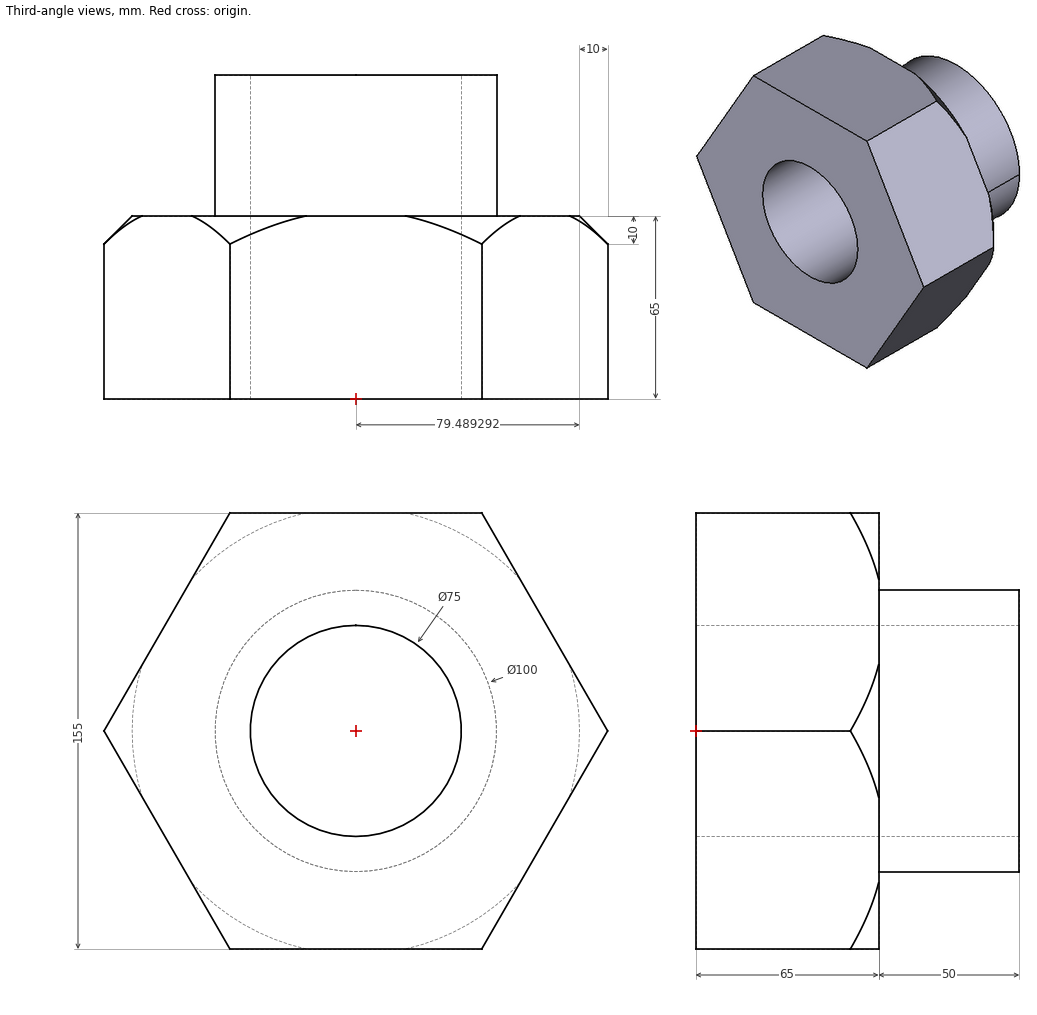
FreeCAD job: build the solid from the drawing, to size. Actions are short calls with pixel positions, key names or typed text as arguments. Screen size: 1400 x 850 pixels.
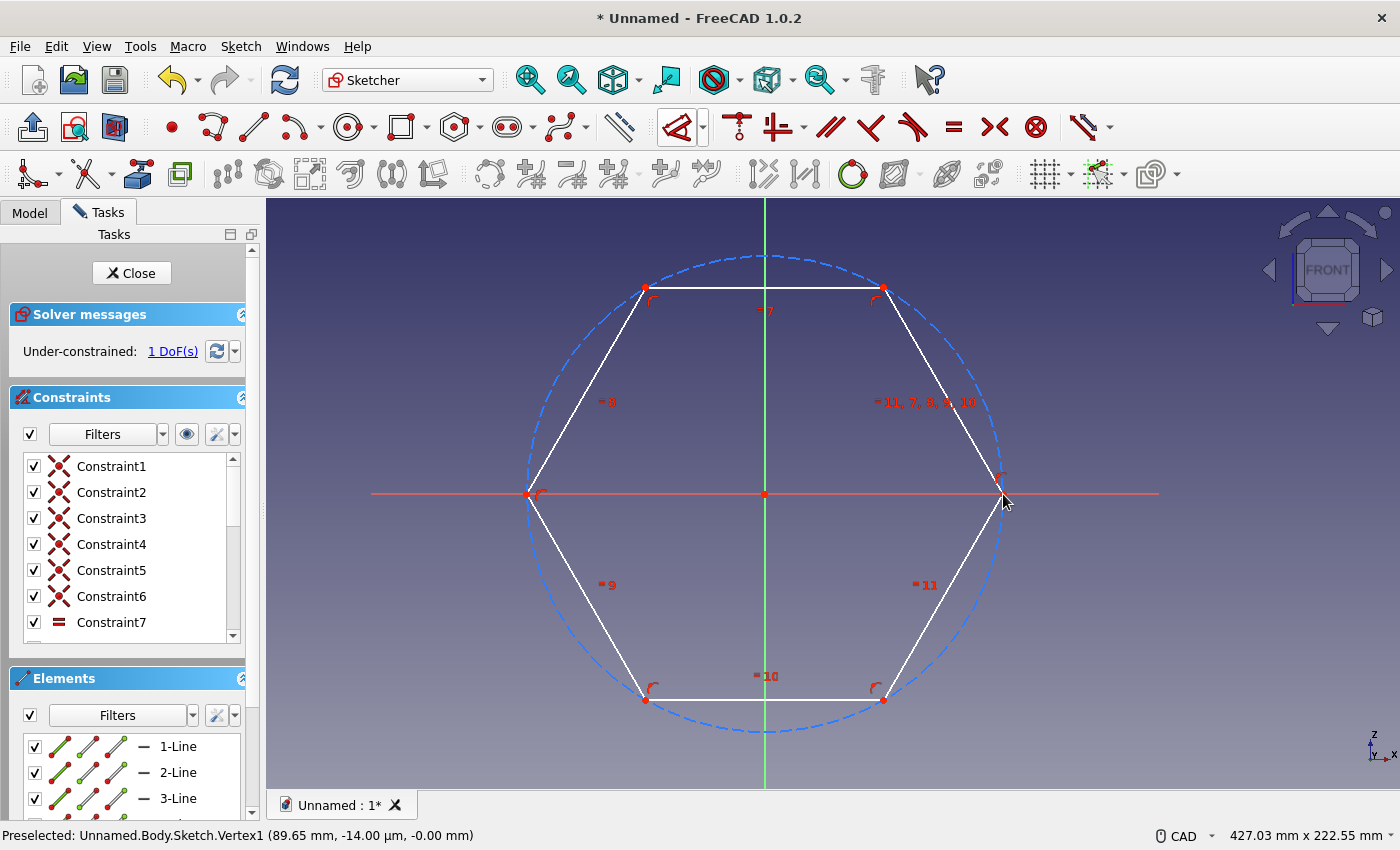
click(646, 700)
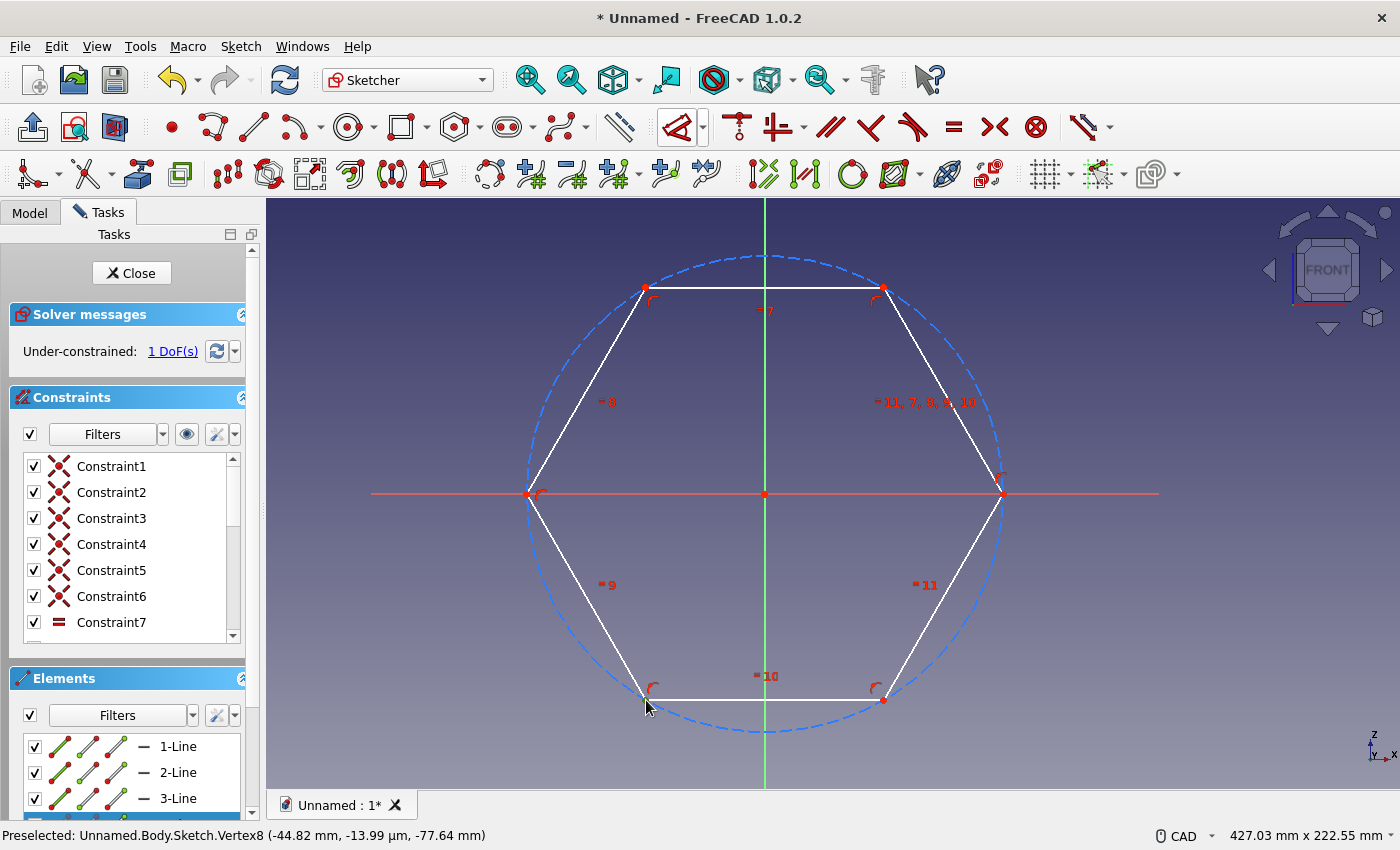
click(884, 288)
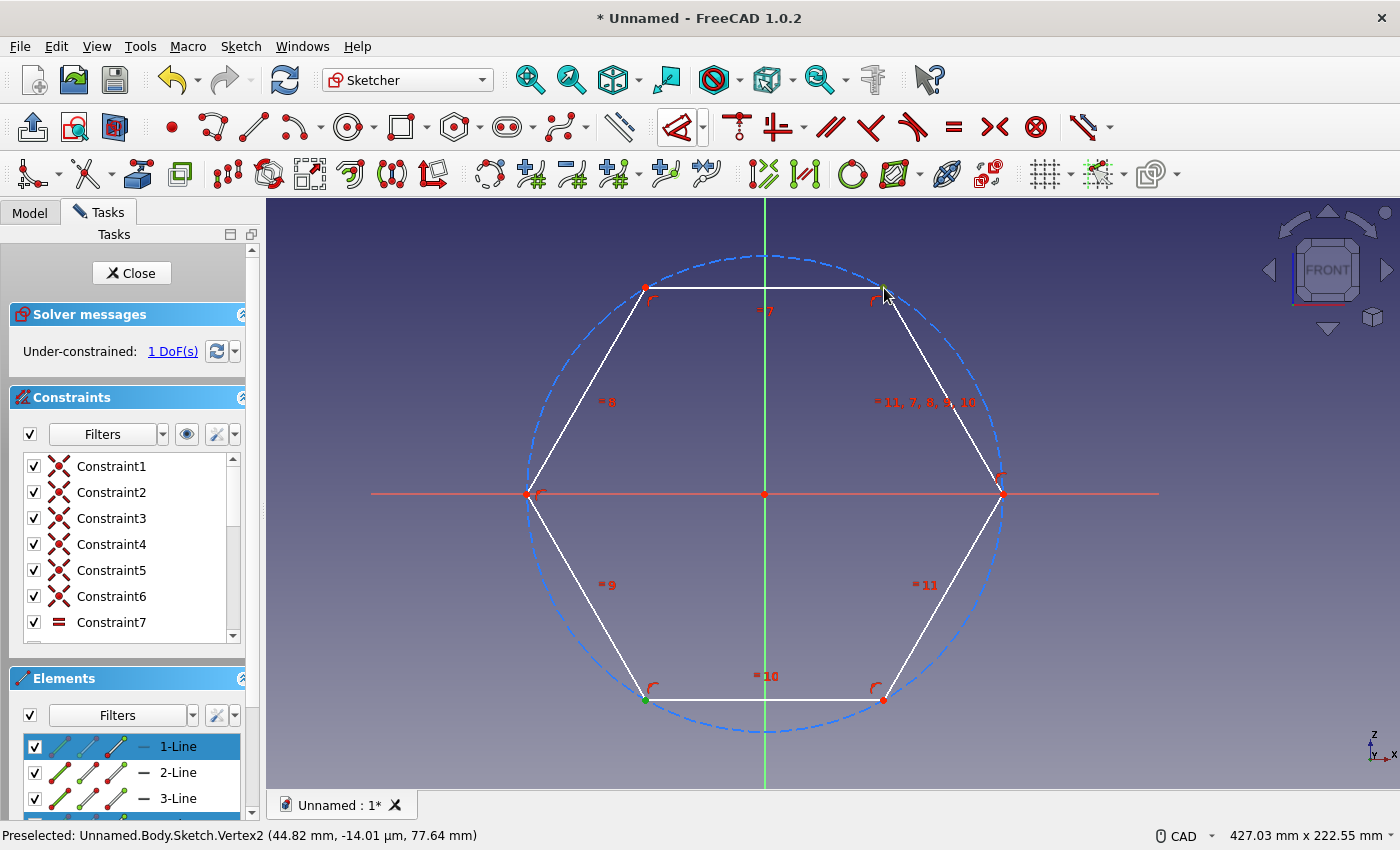
click(702, 128)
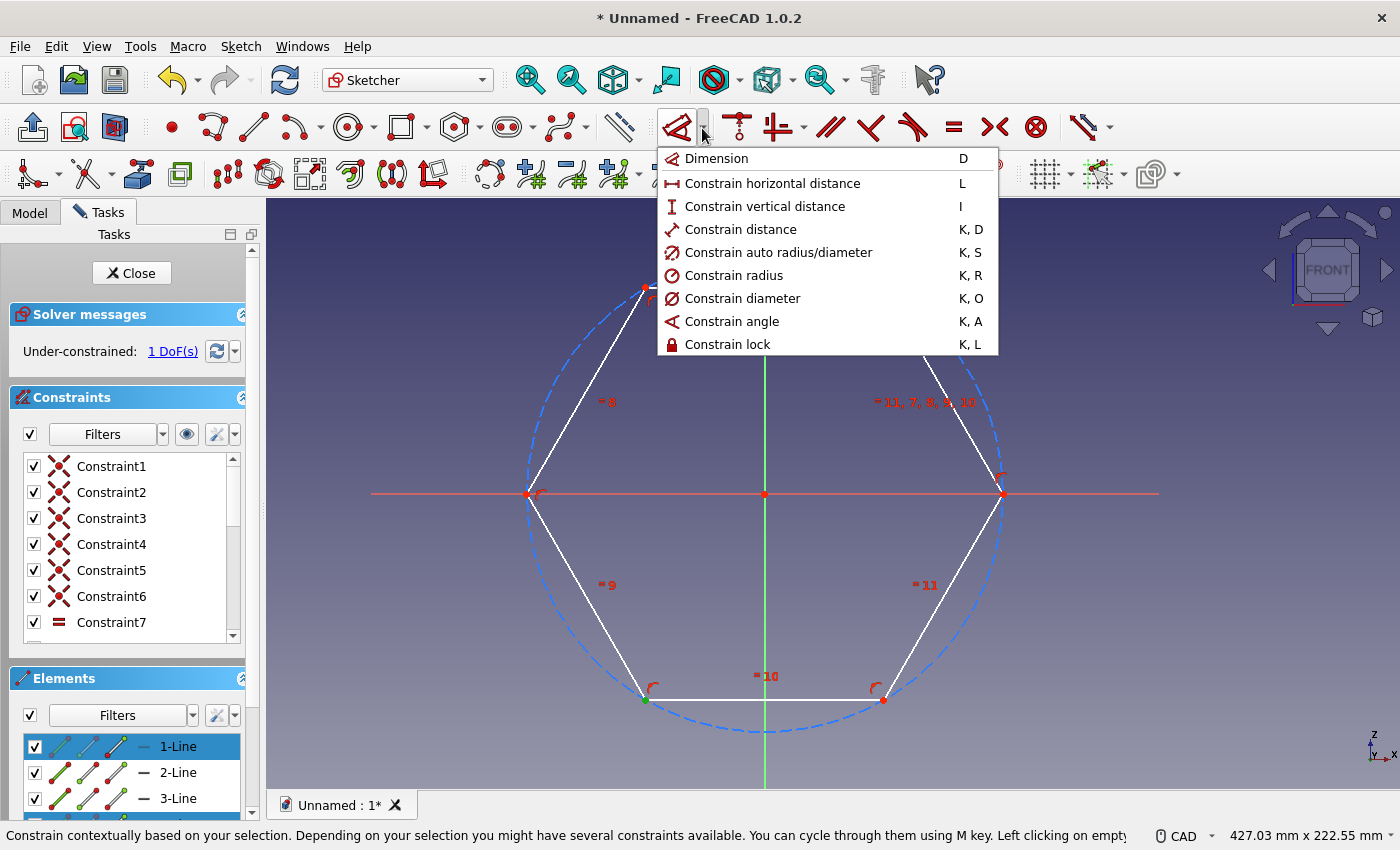
click(828, 206)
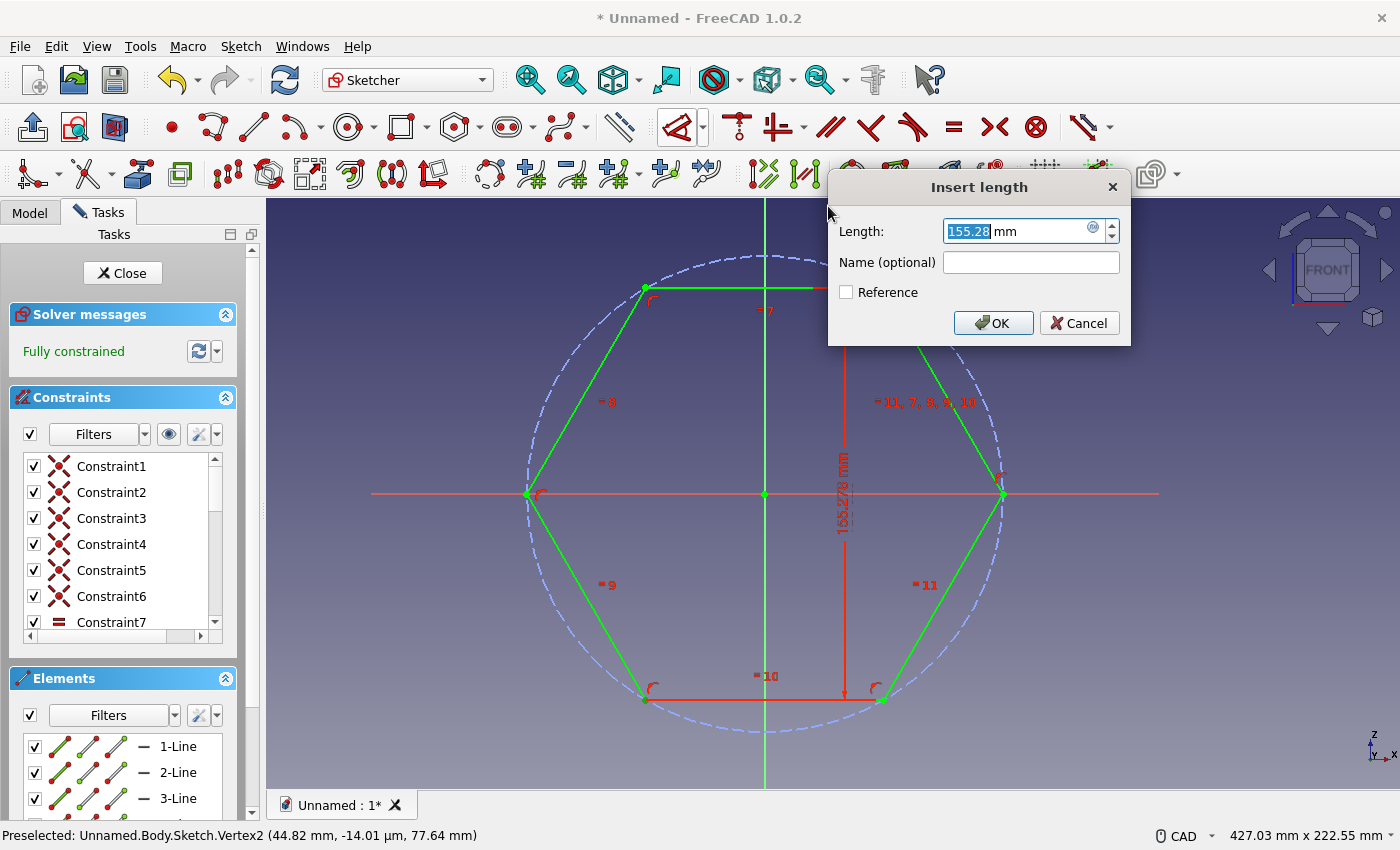
text(155)
key(Return)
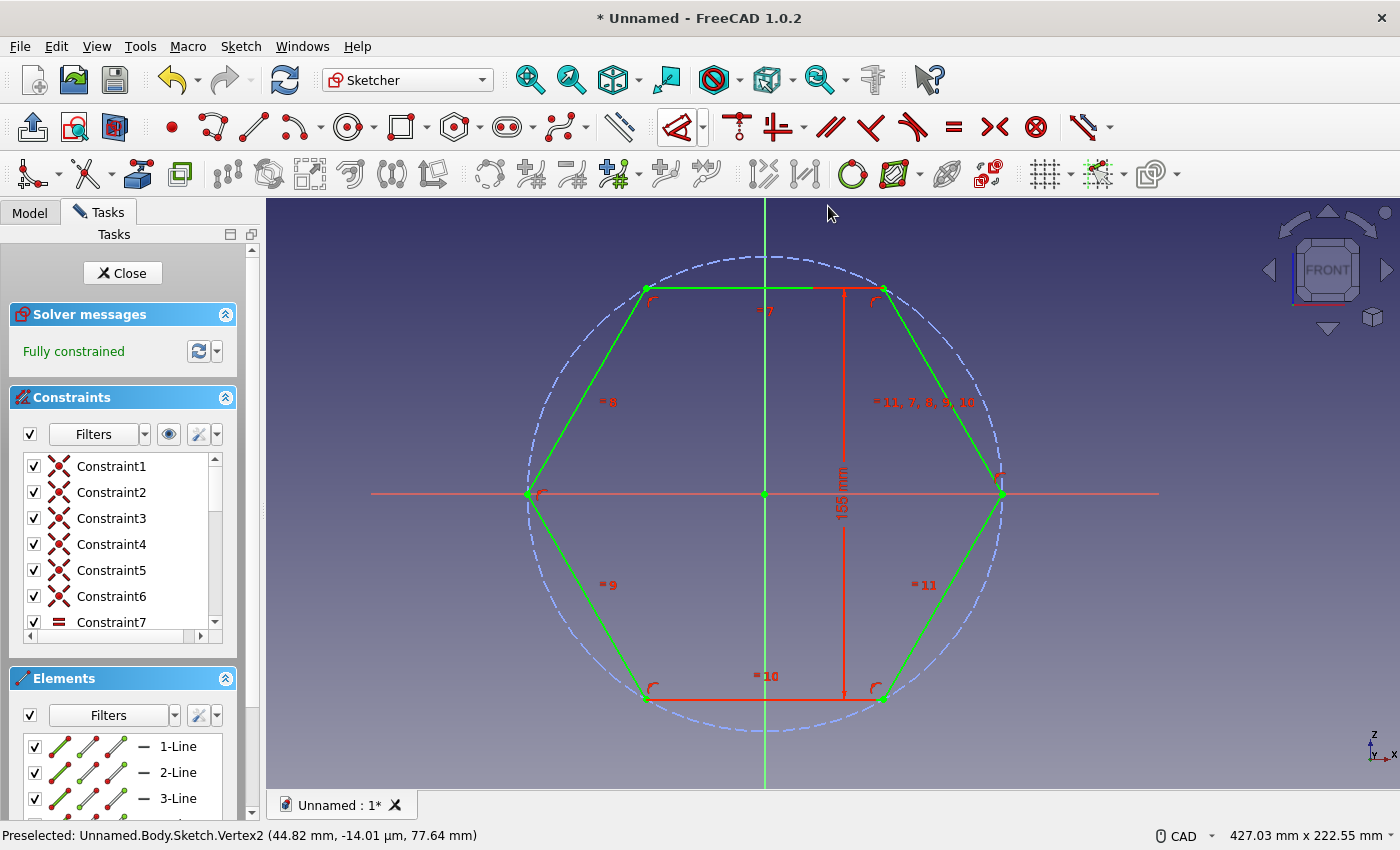
click(123, 273)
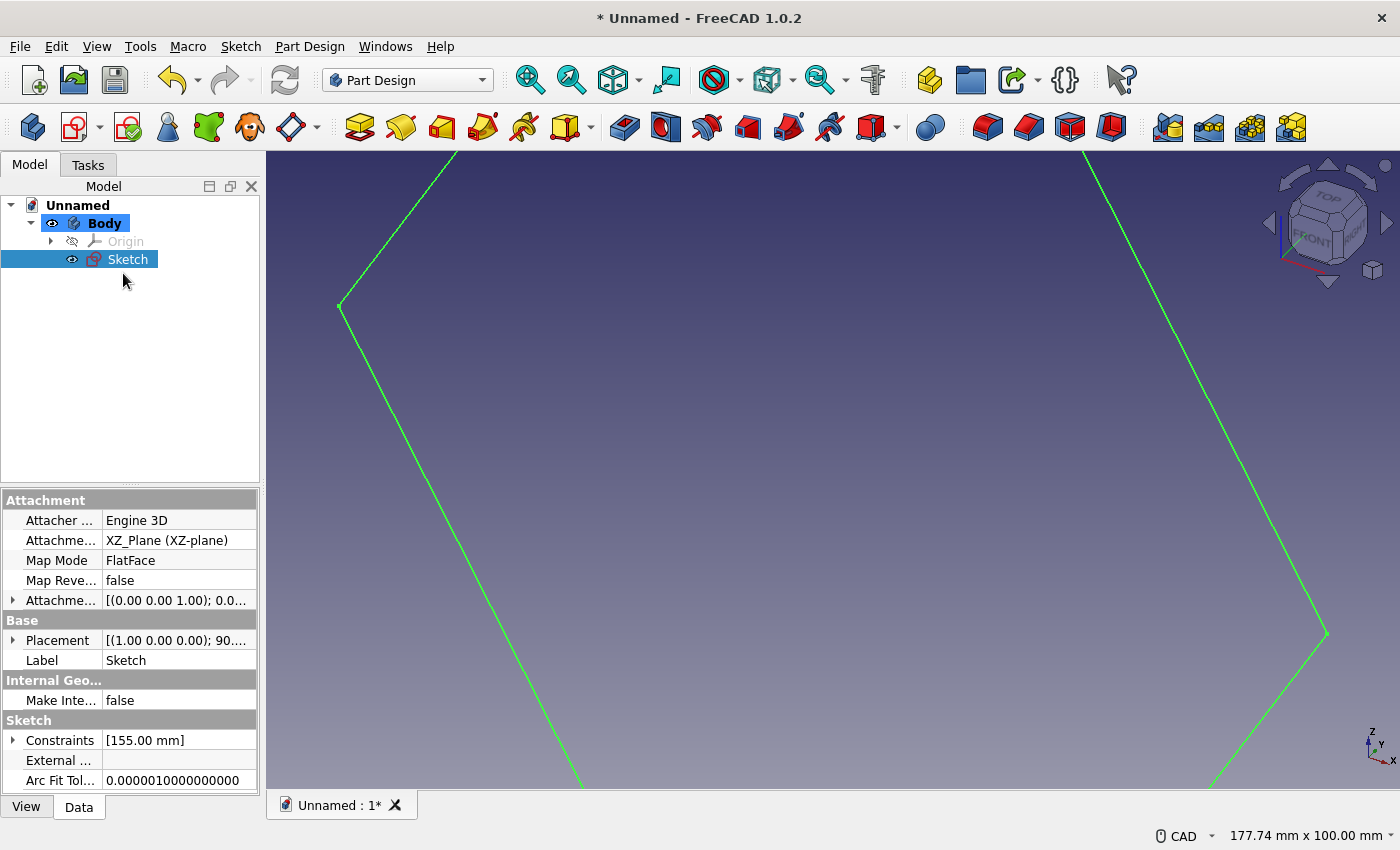
click(360, 128)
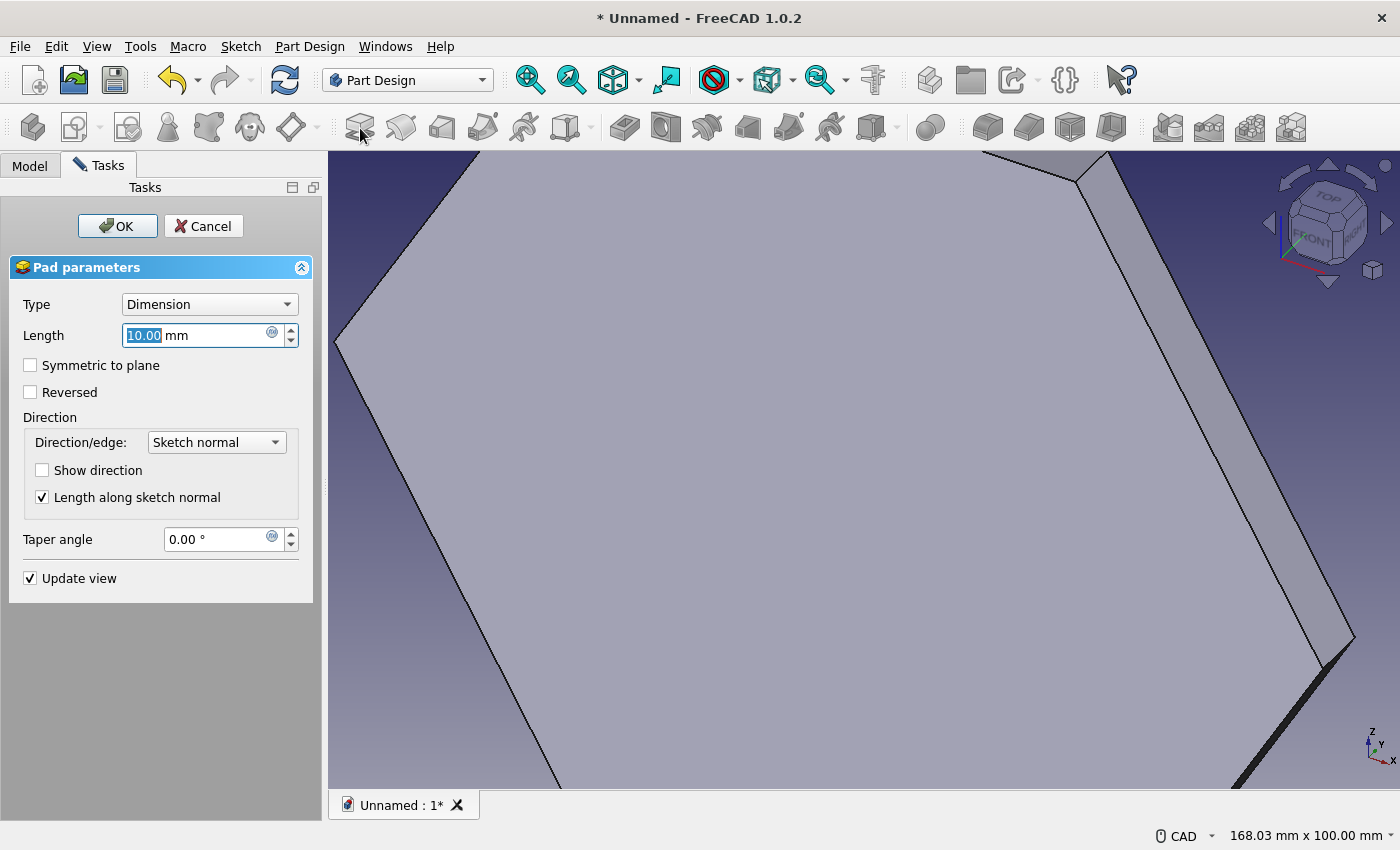
text(65)
key(Tab)